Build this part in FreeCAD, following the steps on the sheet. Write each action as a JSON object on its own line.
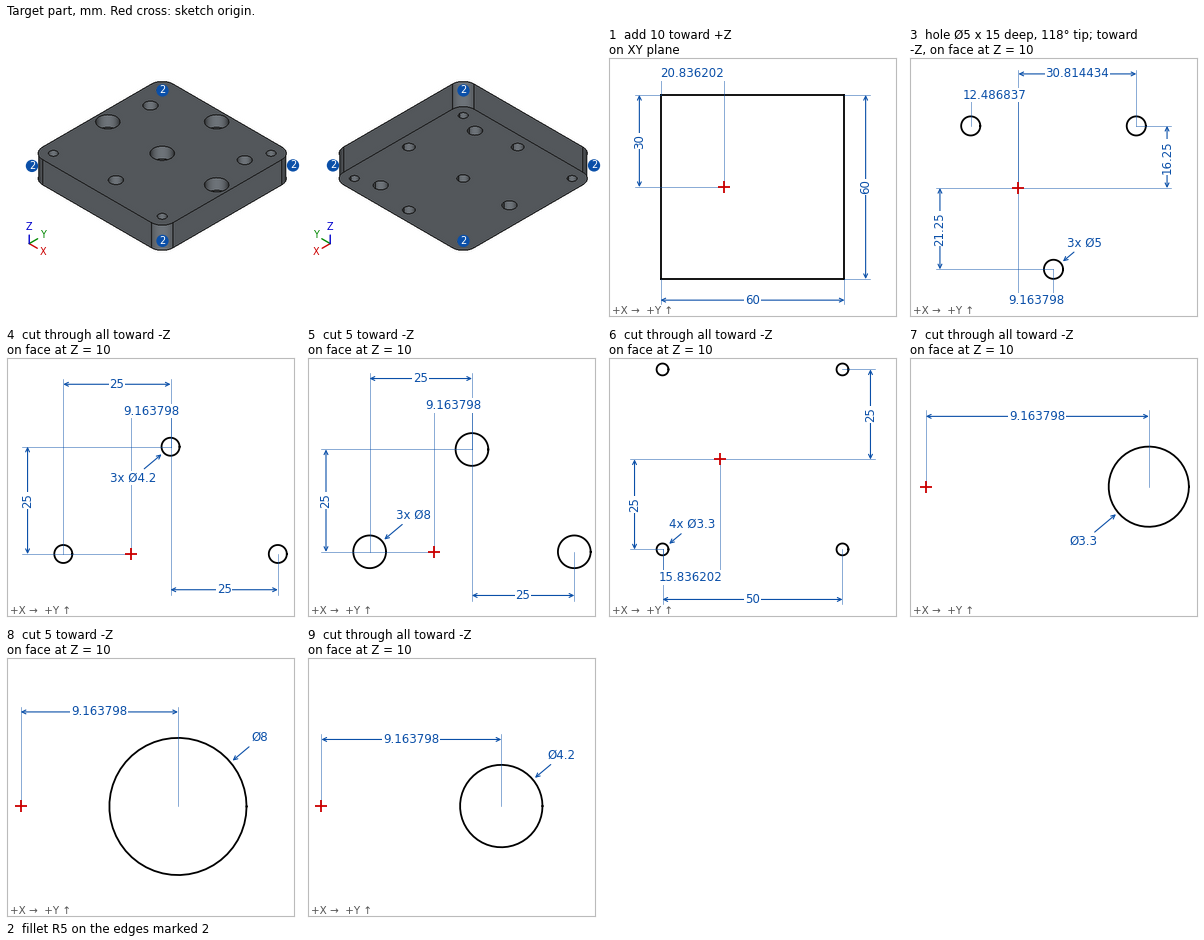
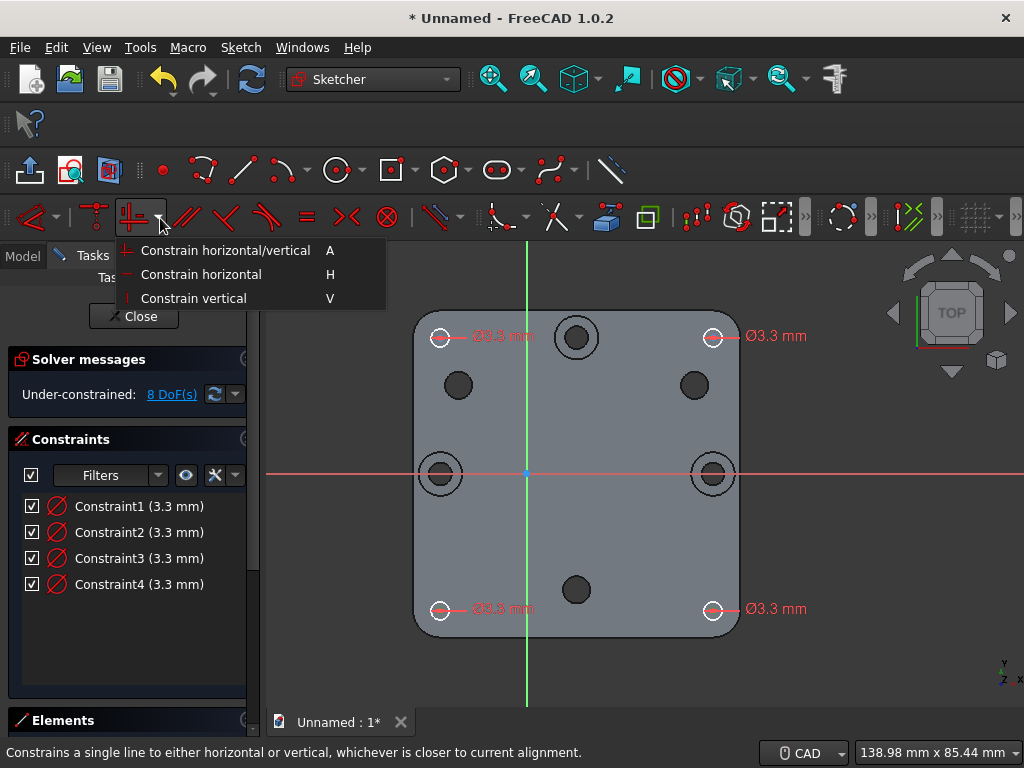
{"action": "left_click", "coordinate": [251, 274]}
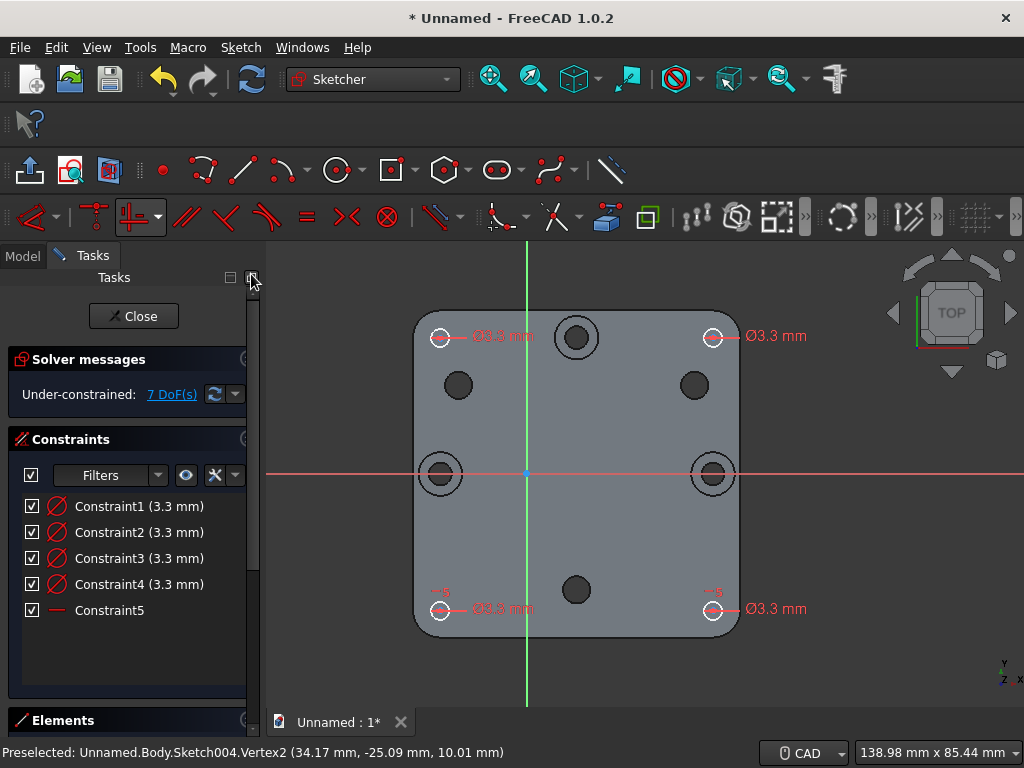
{"action": "left_click", "coordinate": [713, 611]}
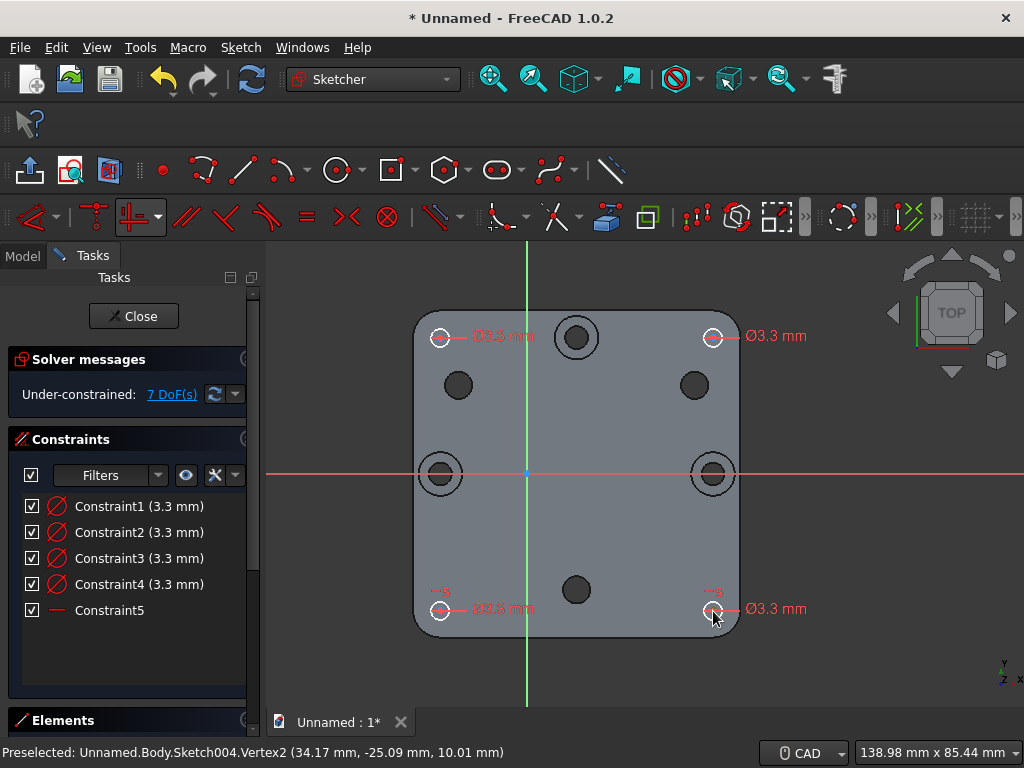
{"action": "left_click", "coordinate": [713, 338]}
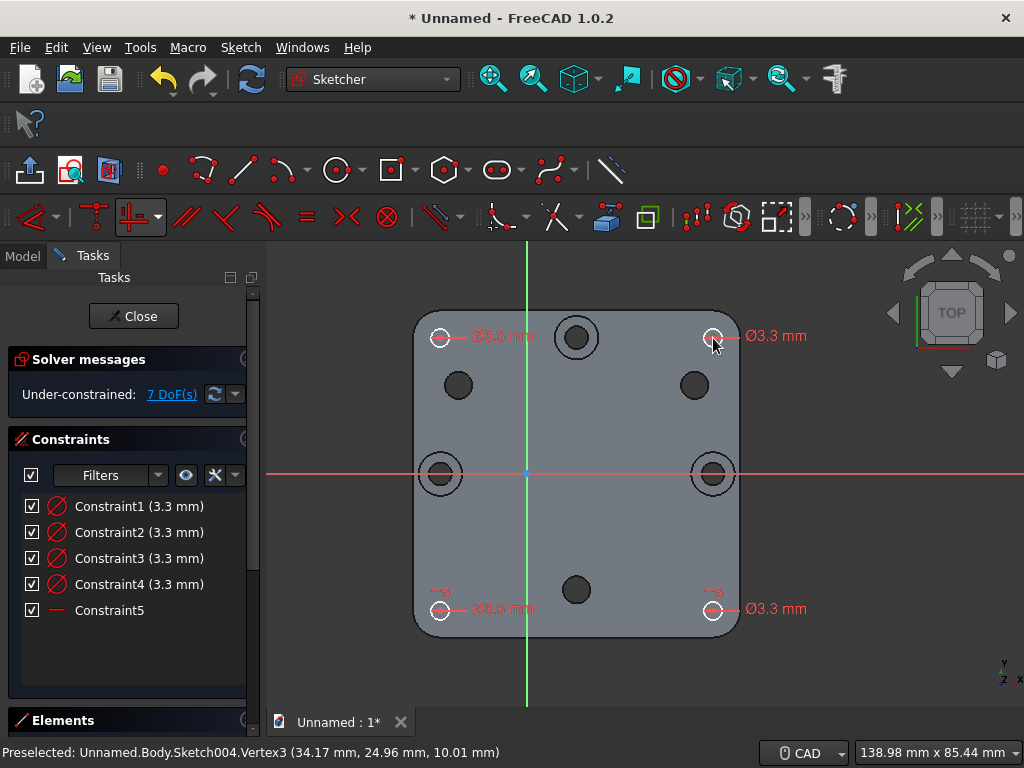
{"action": "key", "text": "v"}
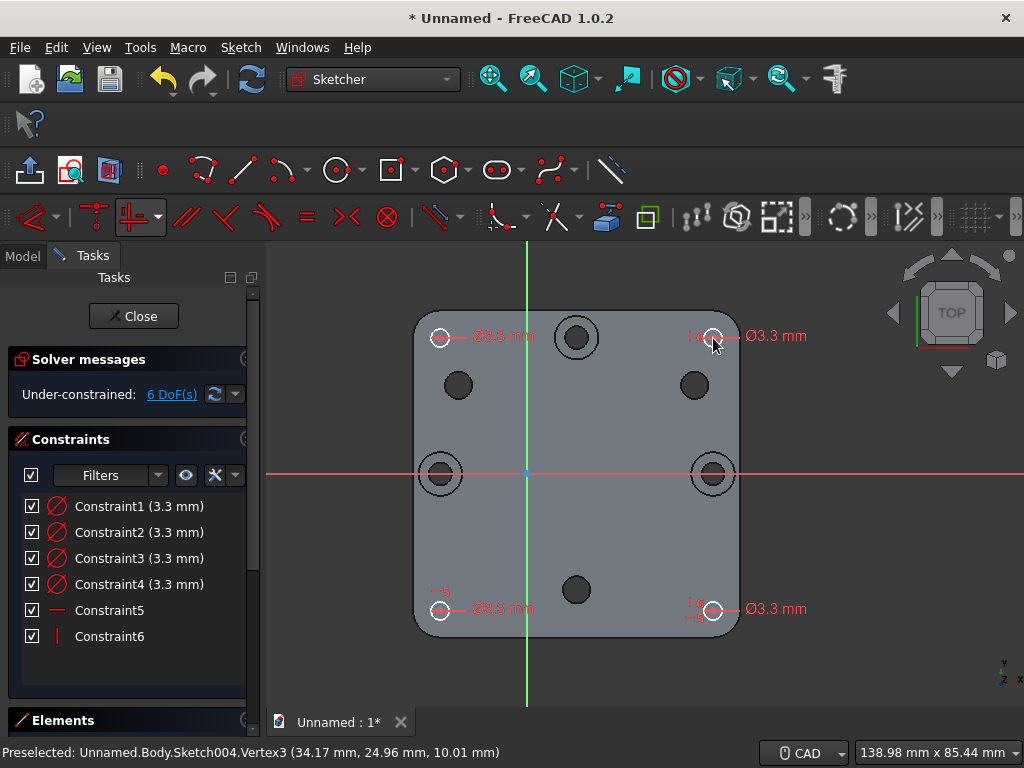
{"action": "left_click", "coordinate": [440, 611]}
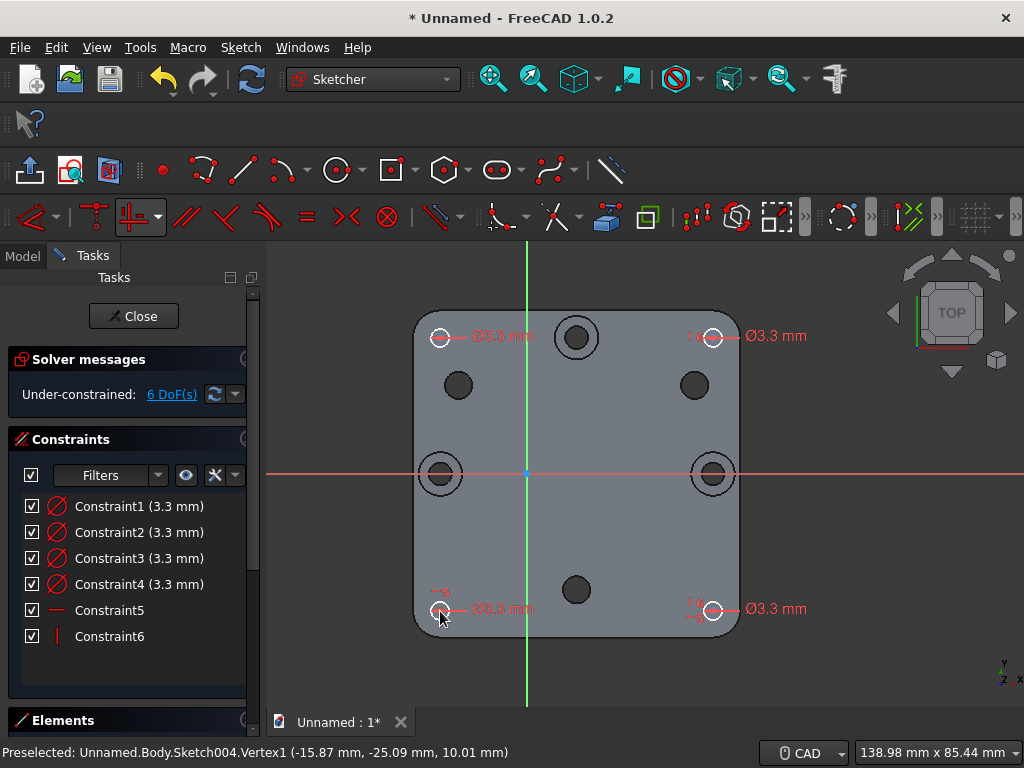
{"action": "left_click", "coordinate": [440, 338]}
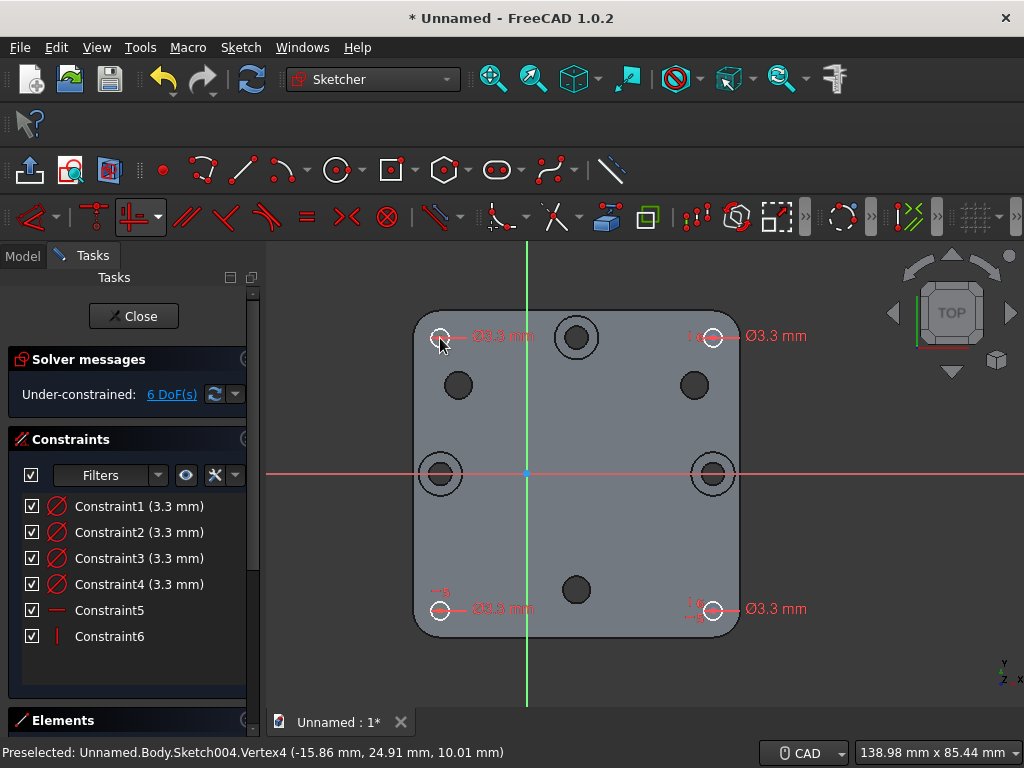
{"action": "key", "text": "v"}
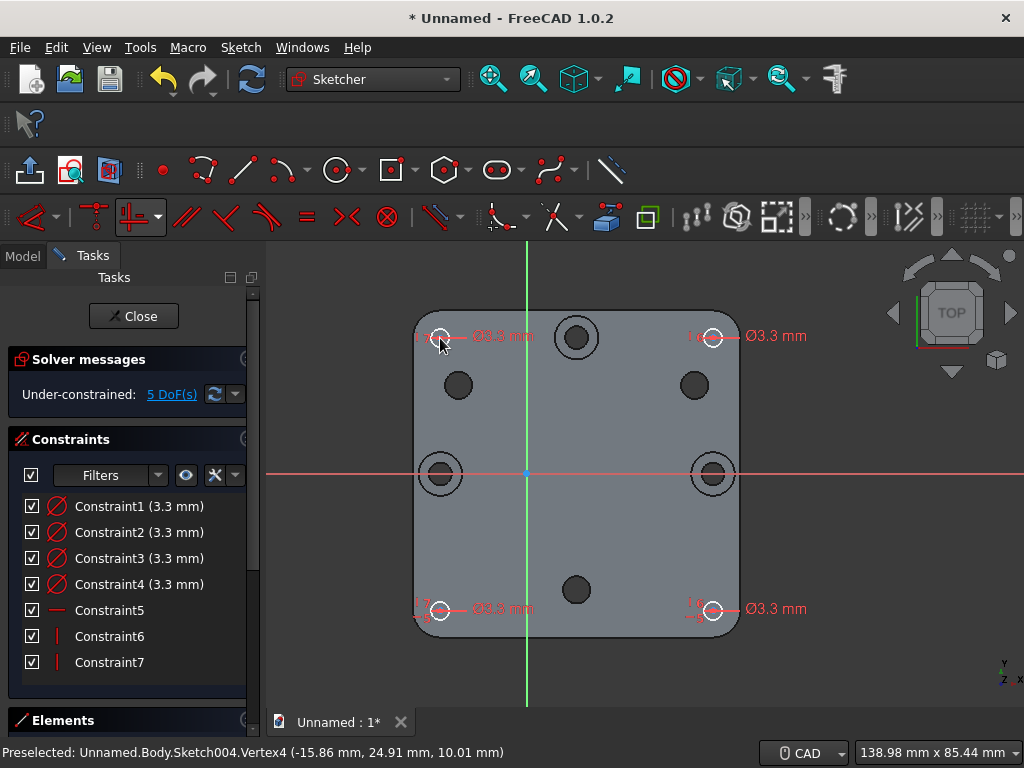
{"action": "left_click", "coordinate": [713, 338]}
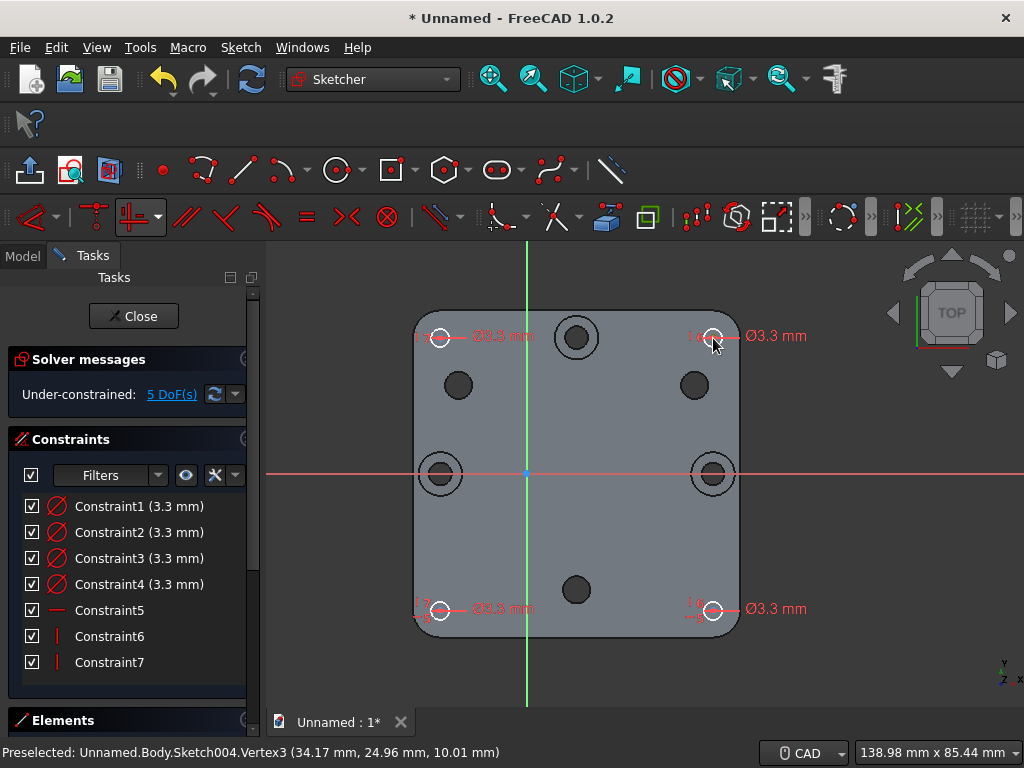
{"action": "left_click", "coordinate": [440, 338]}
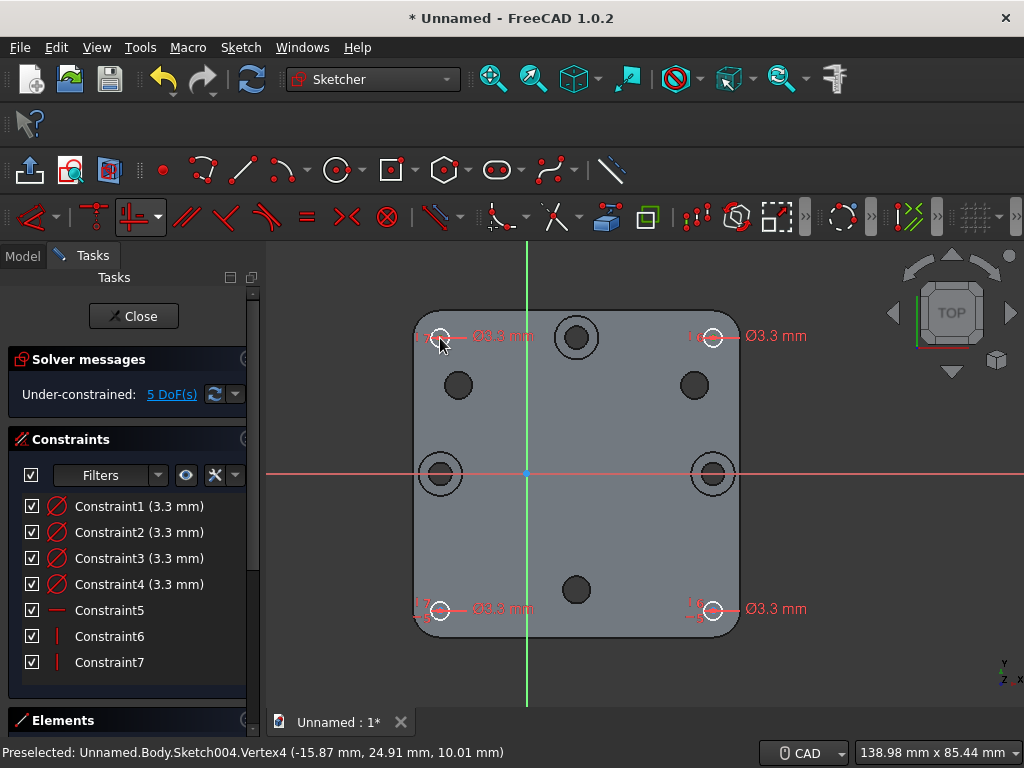
{"action": "left_click", "coordinate": [160, 218]}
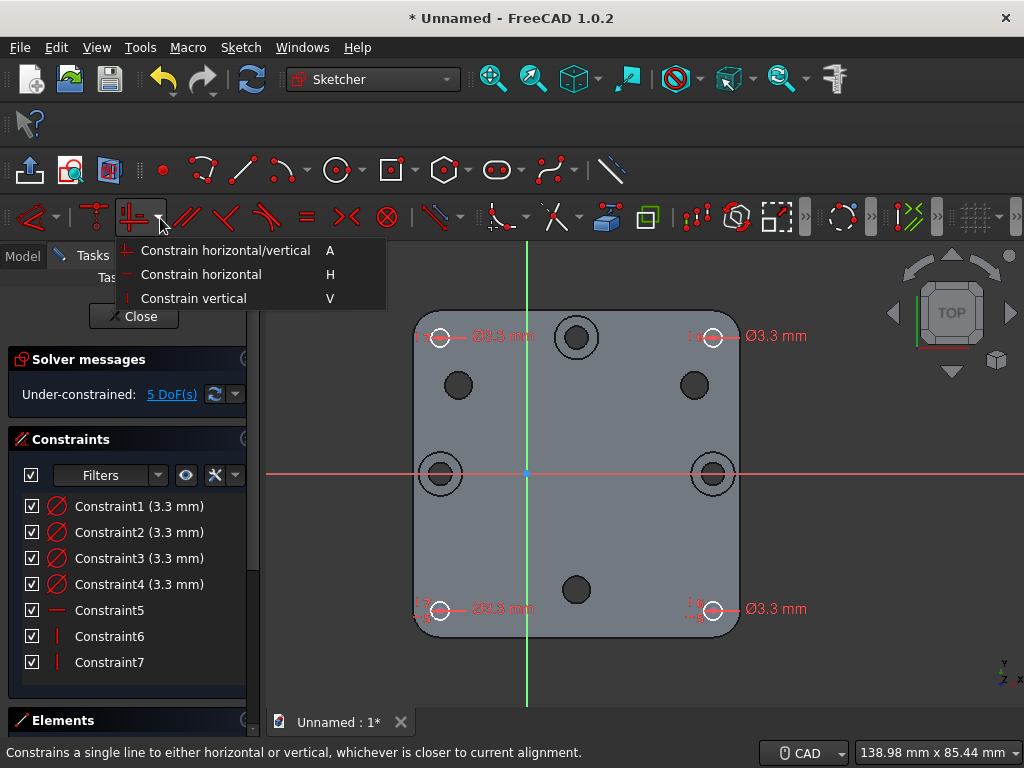
{"action": "left_click", "coordinate": [251, 274]}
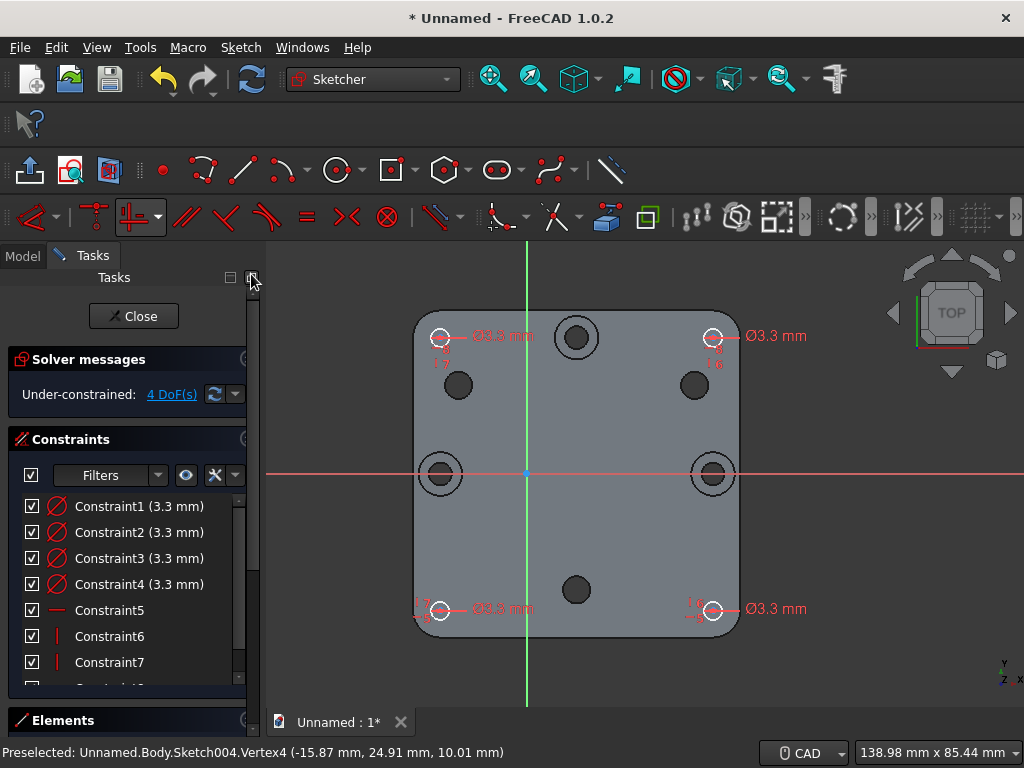
{"action": "left_click", "coordinate": [32, 218]}